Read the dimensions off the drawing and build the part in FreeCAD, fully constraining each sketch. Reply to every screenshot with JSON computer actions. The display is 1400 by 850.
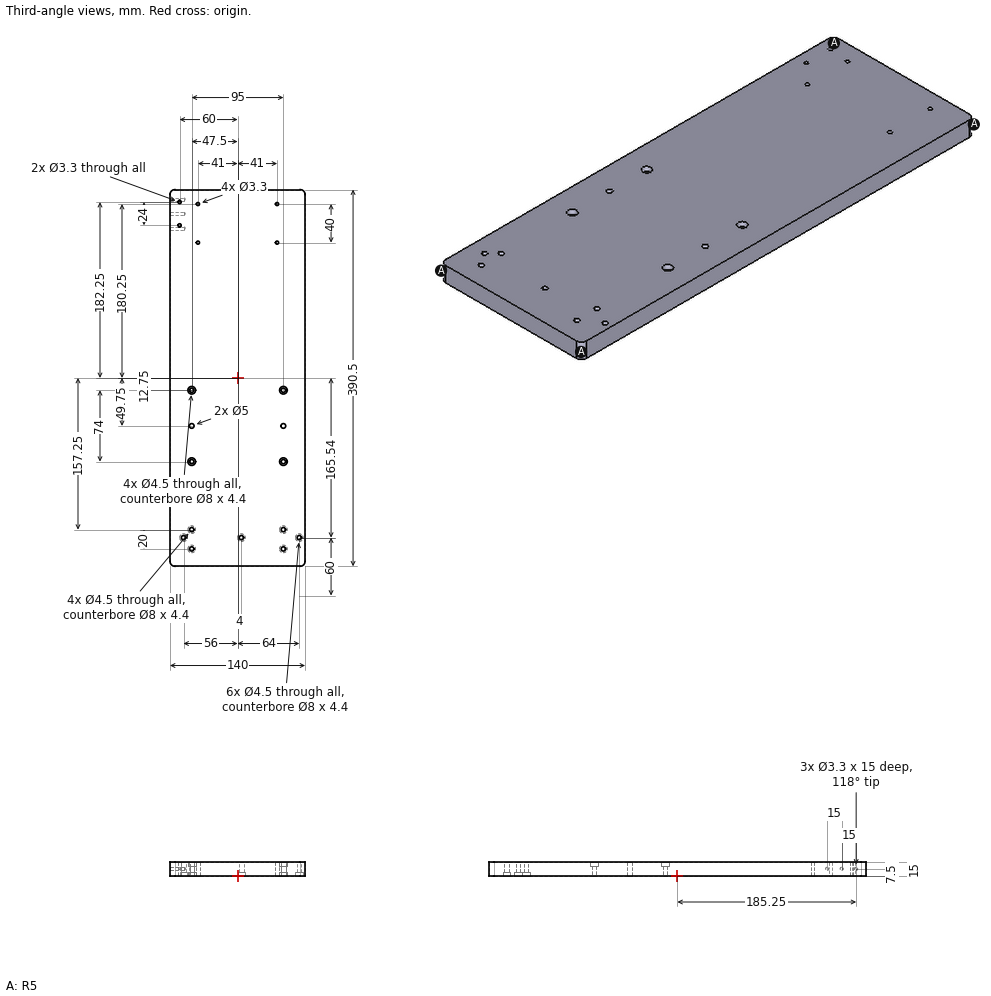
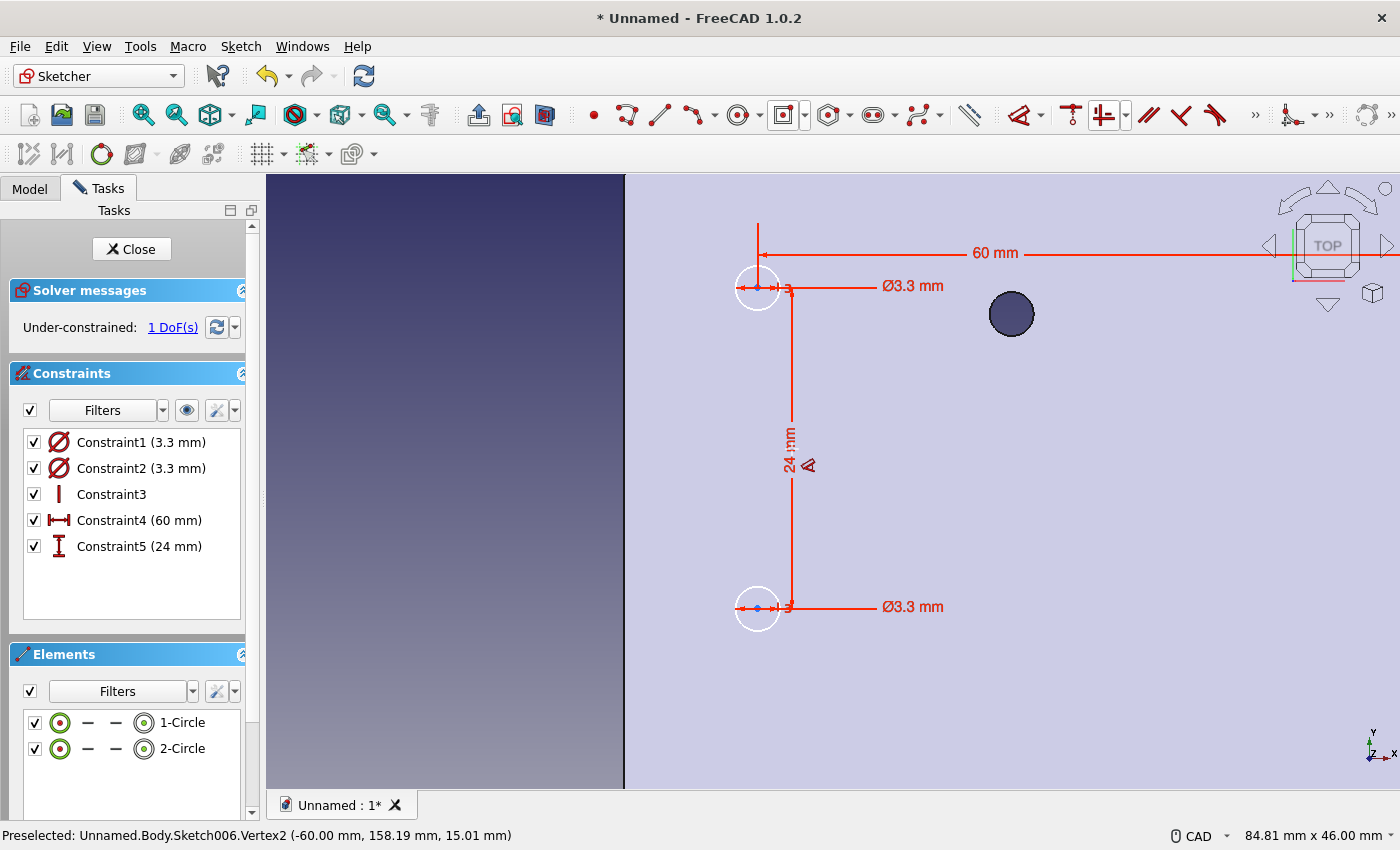
{"action": "left_click", "coordinate": [758, 288]}
{"action": "left_click", "coordinate": [724, 525]}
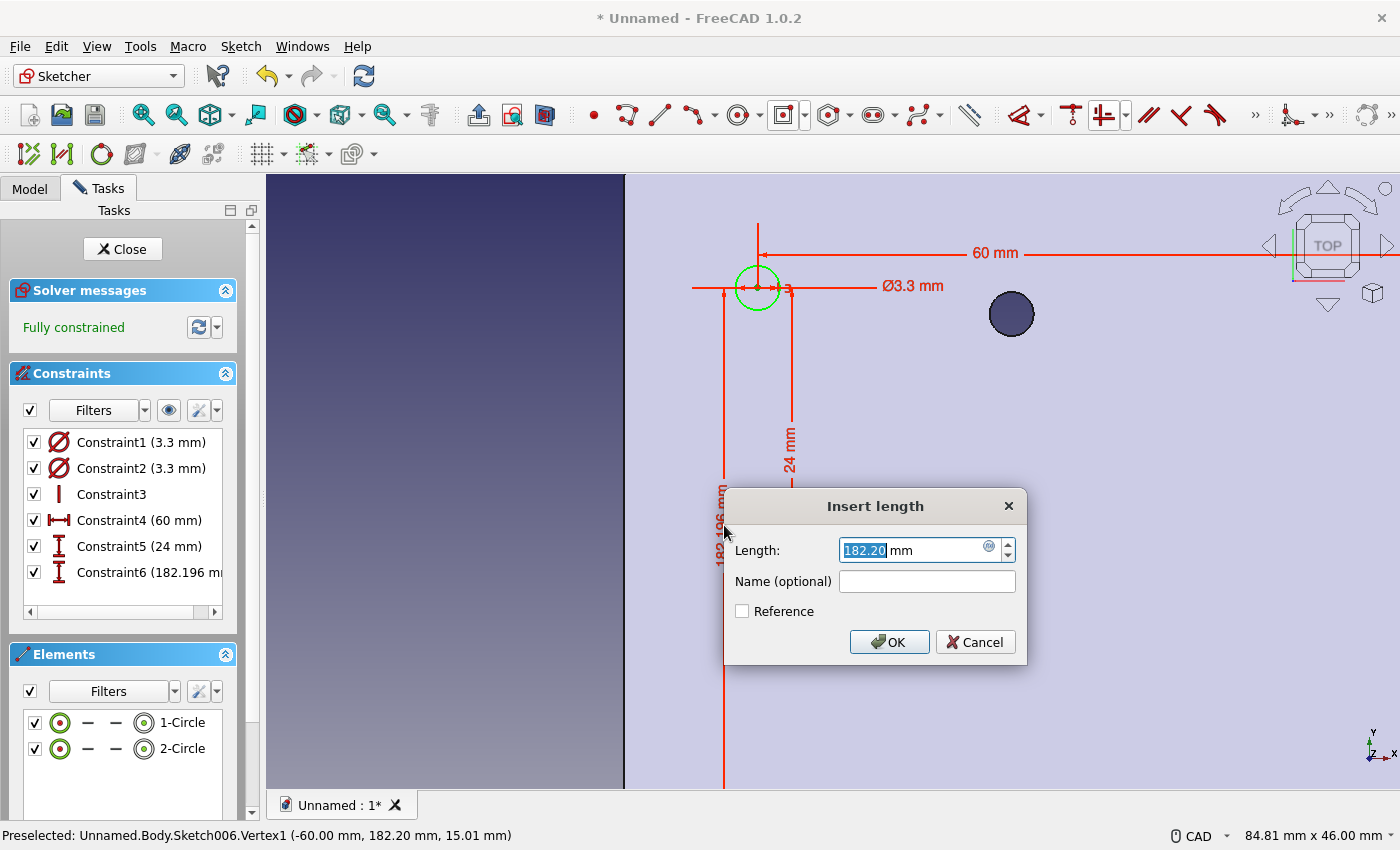
{"action": "type", "text": "182.25"}
{"action": "key", "text": "Return"}
{"action": "key", "text": "Escape"}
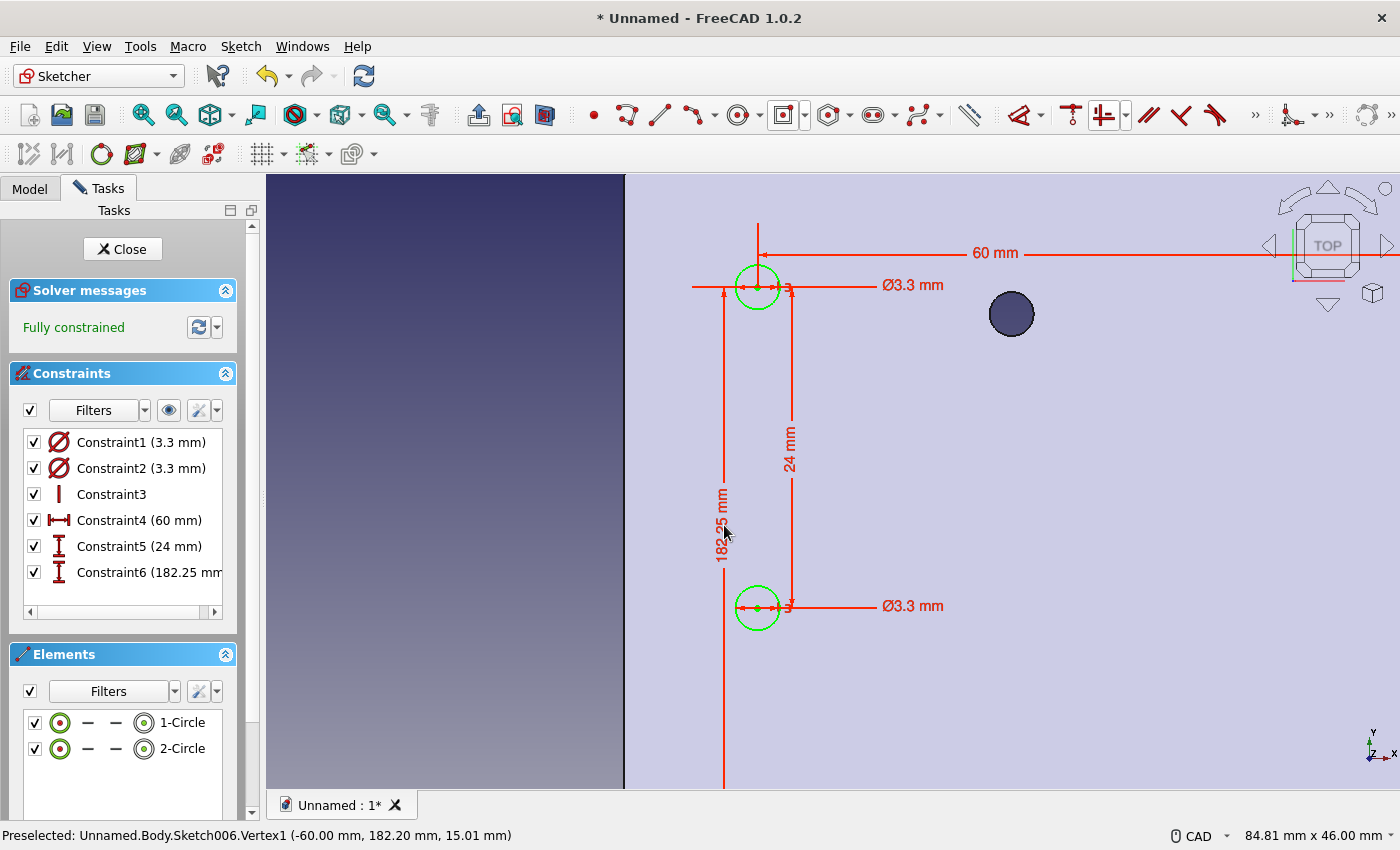
{"action": "left_click", "coordinate": [123, 249]}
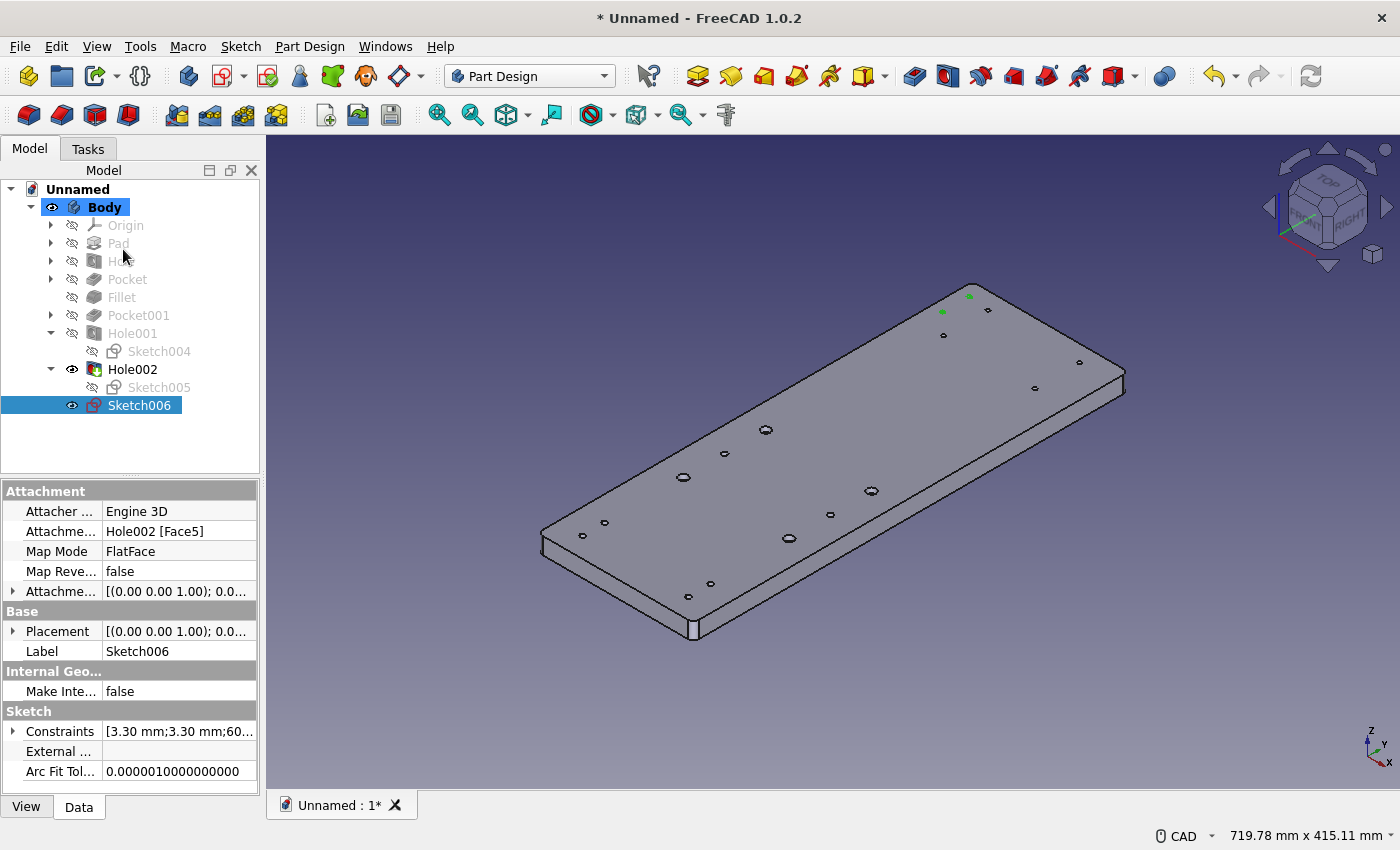
{"action": "left_click", "coordinate": [948, 76]}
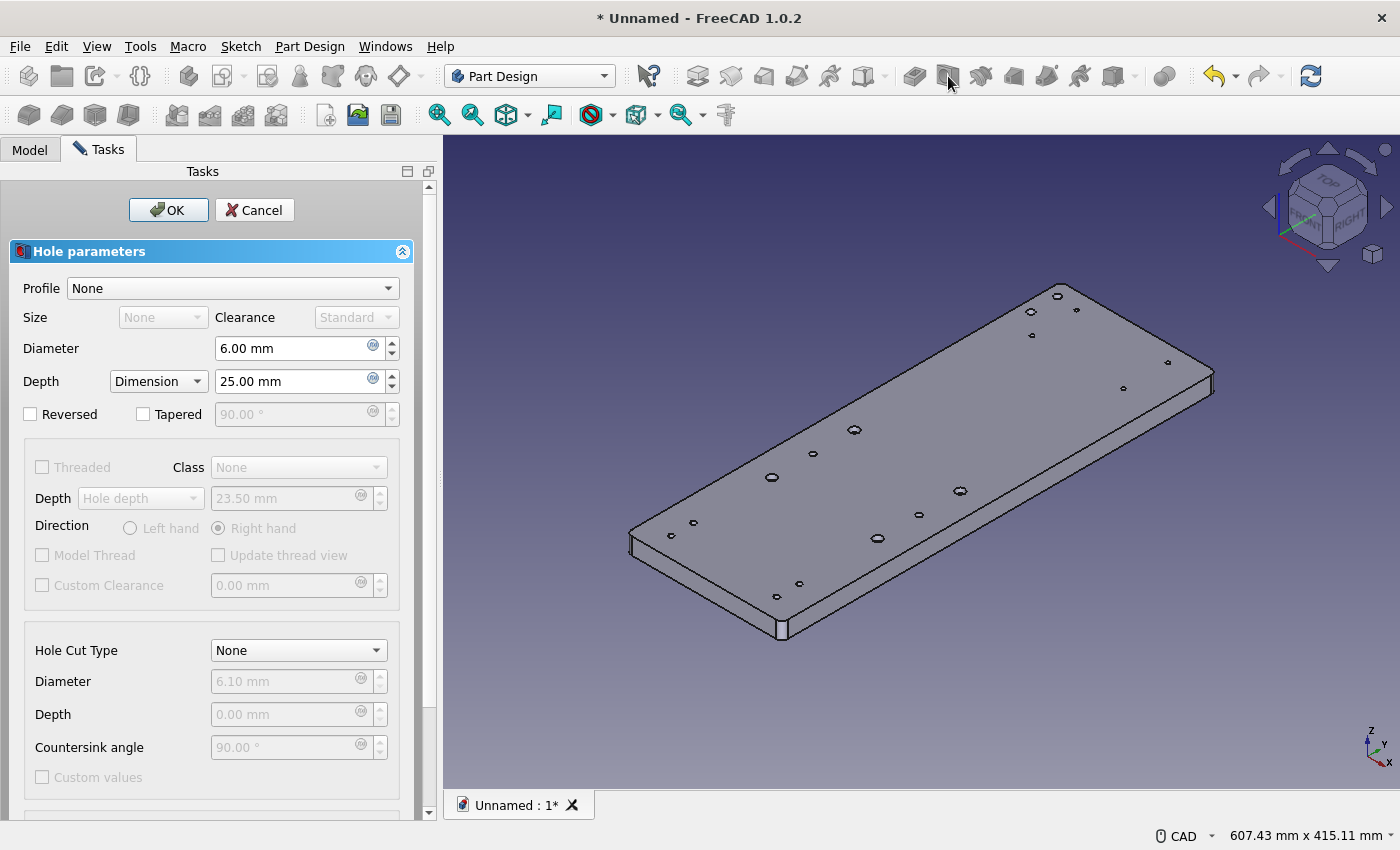
{"action": "triple_click", "coordinate": [300, 348]}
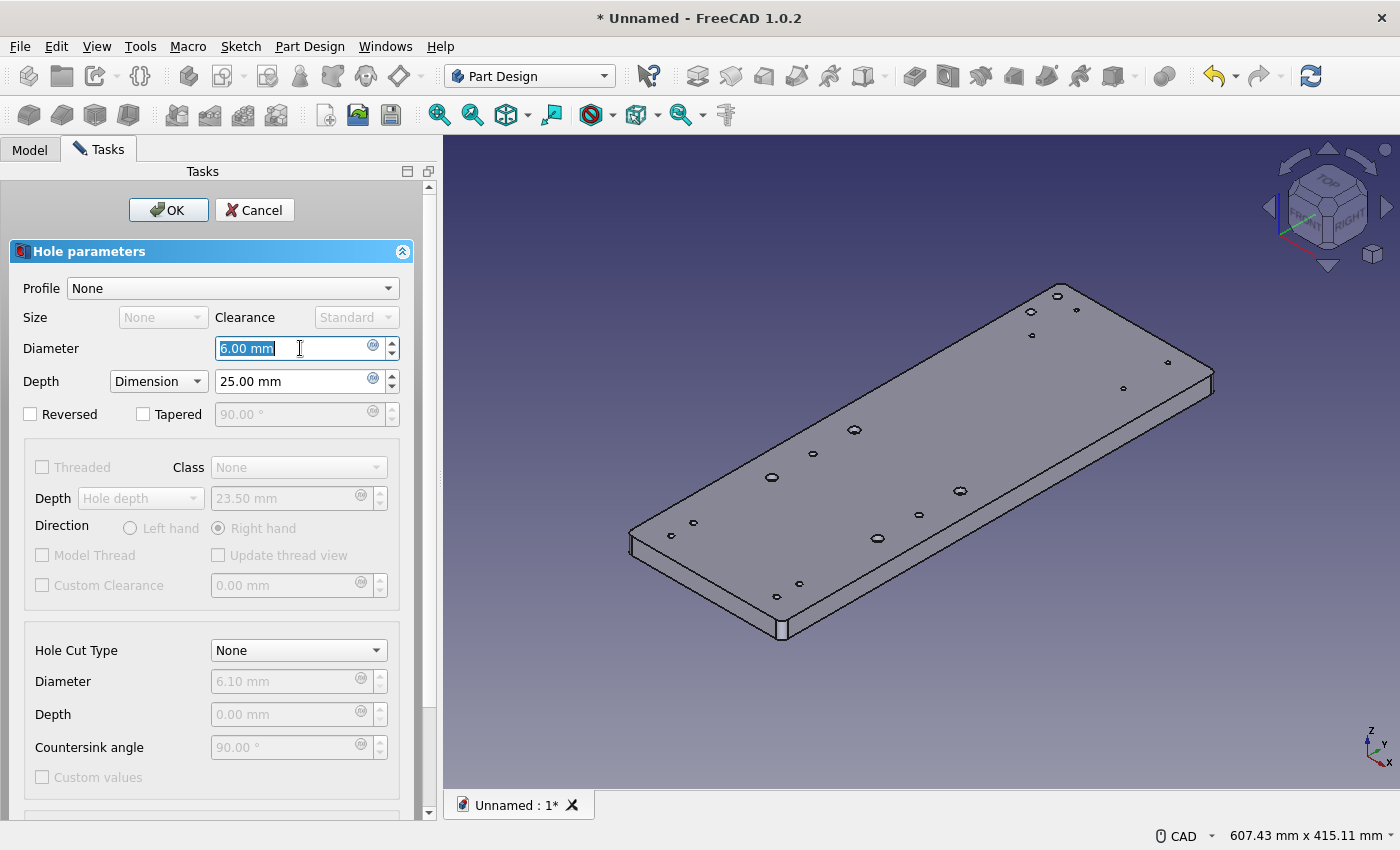
{"action": "type", "text": "3.3"}
{"action": "key", "text": "Tab"}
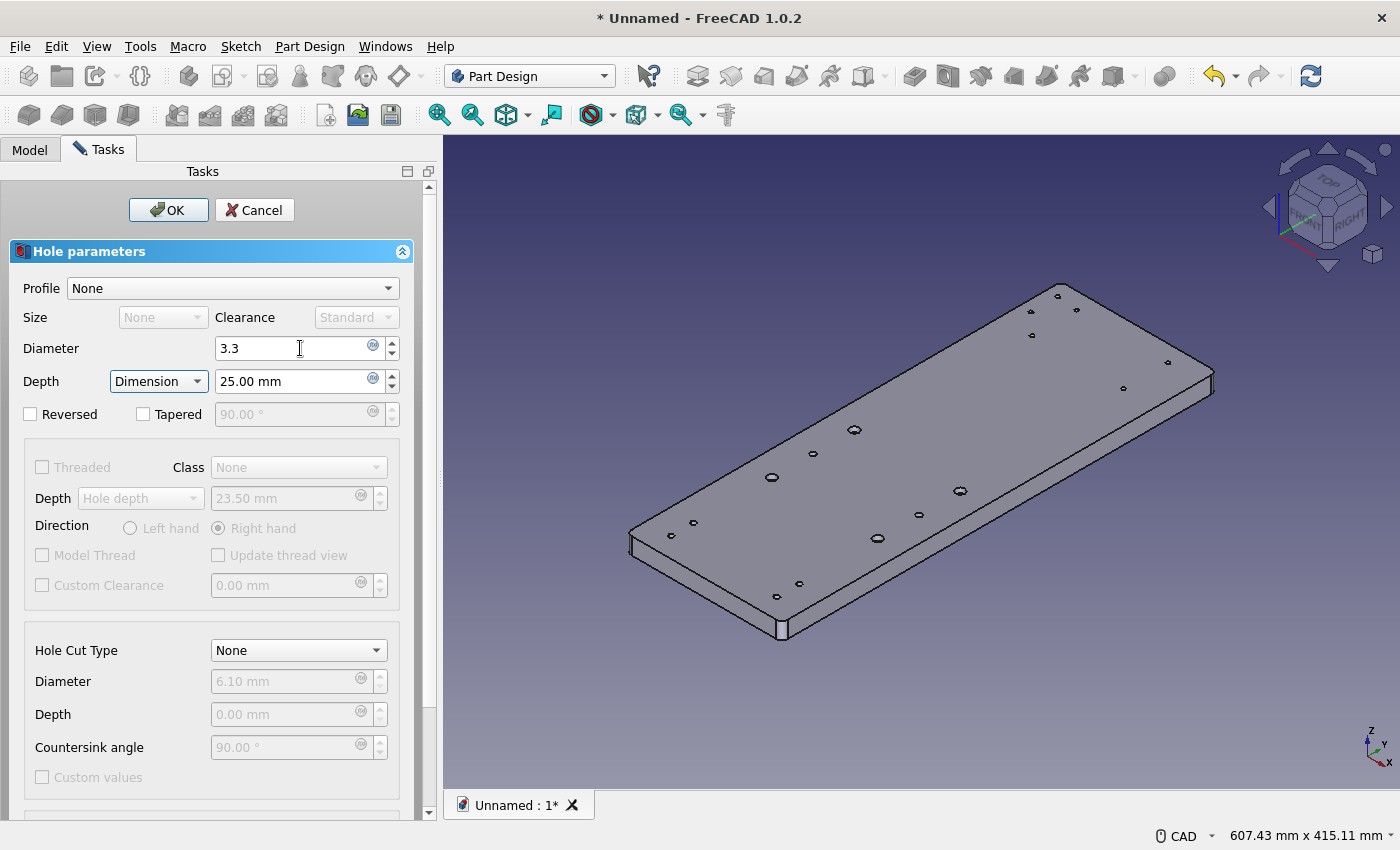
{"action": "left_click", "coordinate": [160, 382]}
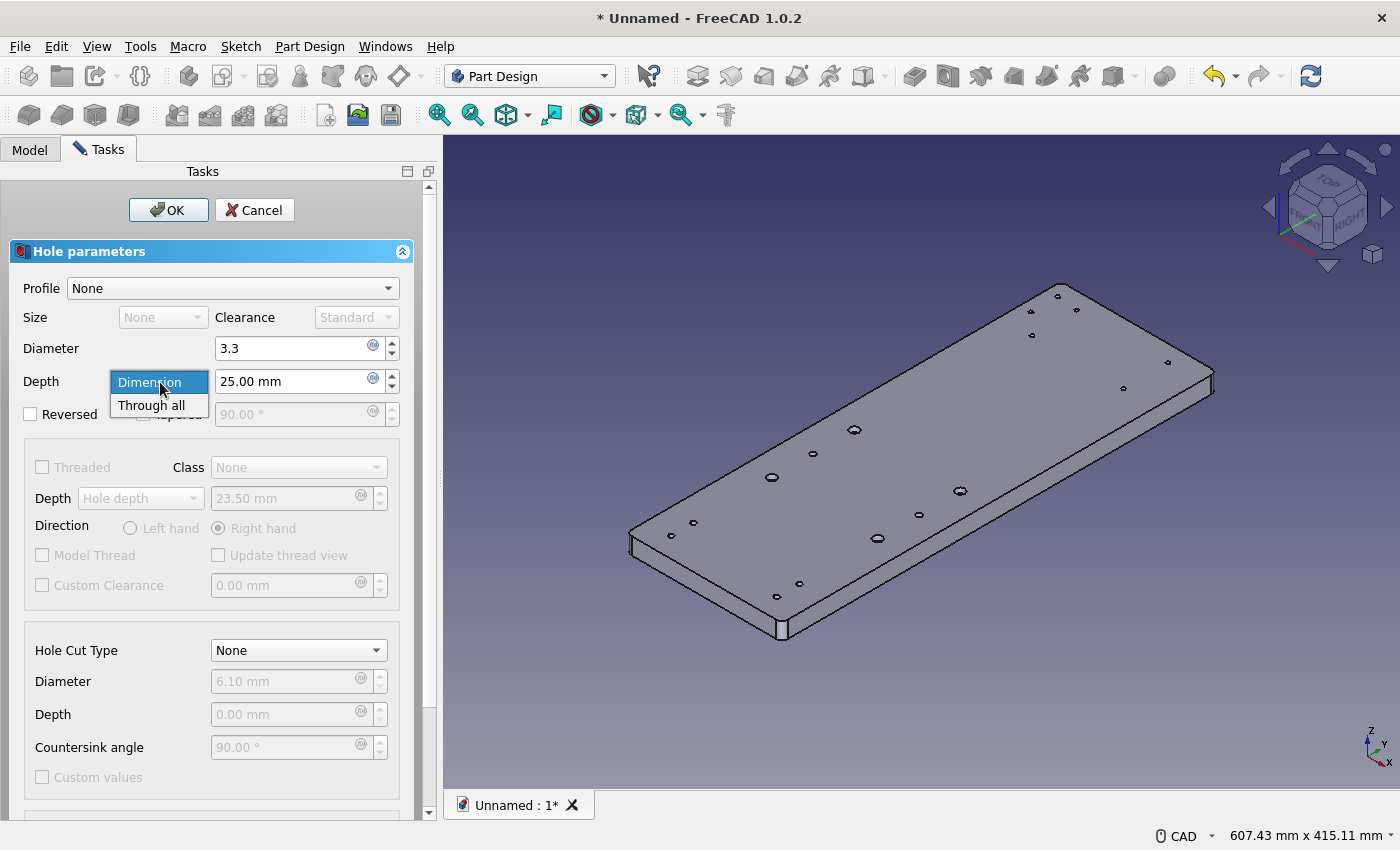
{"action": "left_click", "coordinate": [158, 406]}